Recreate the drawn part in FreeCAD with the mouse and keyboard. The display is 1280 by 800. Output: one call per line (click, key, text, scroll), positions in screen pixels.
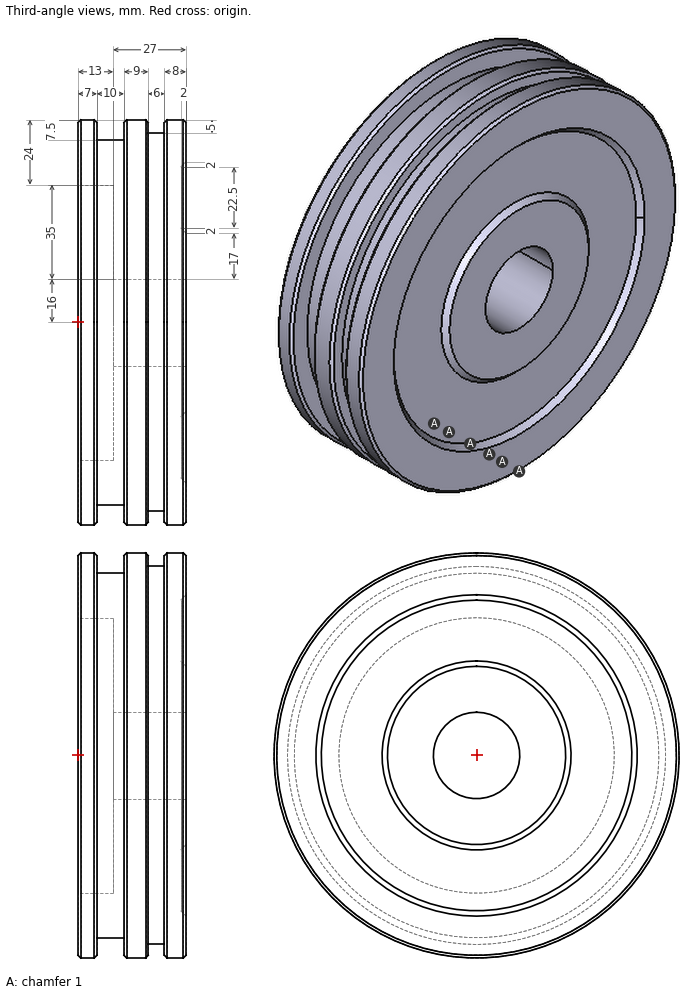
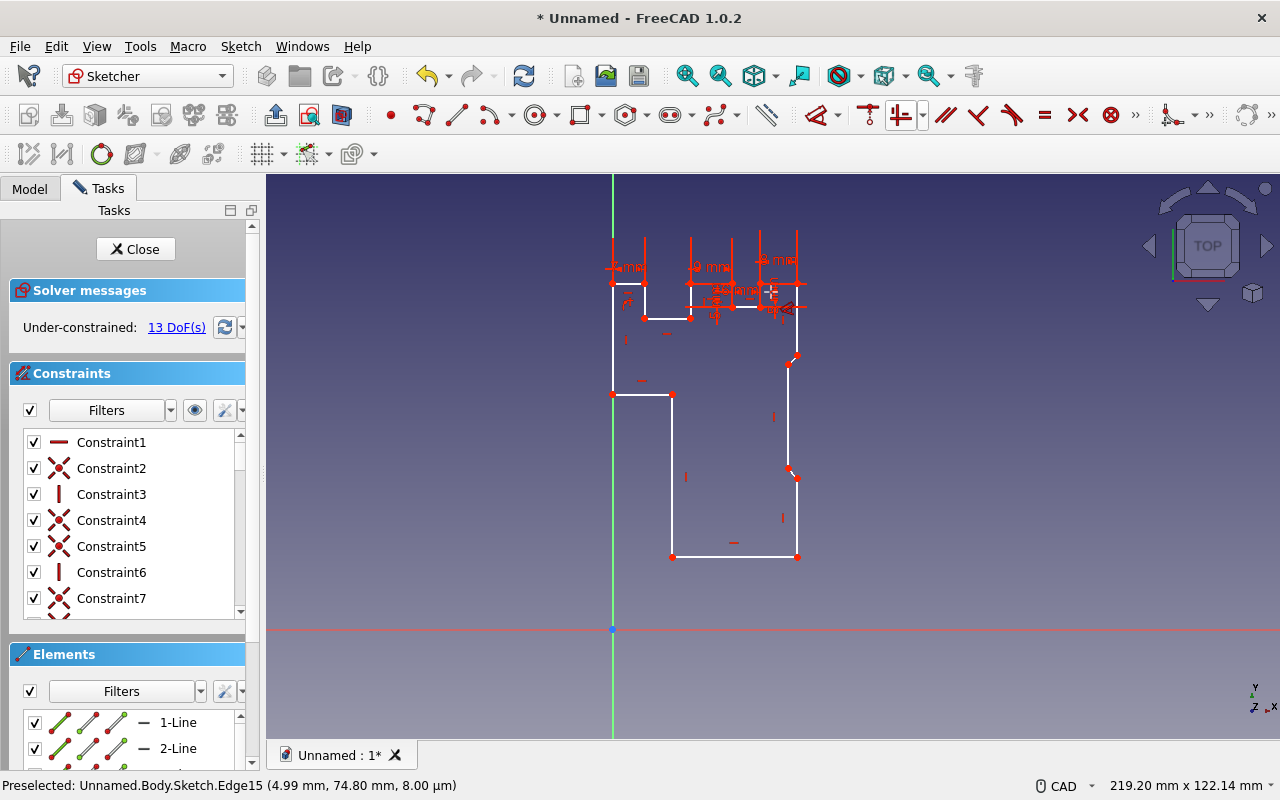
click(710, 557)
click(735, 591)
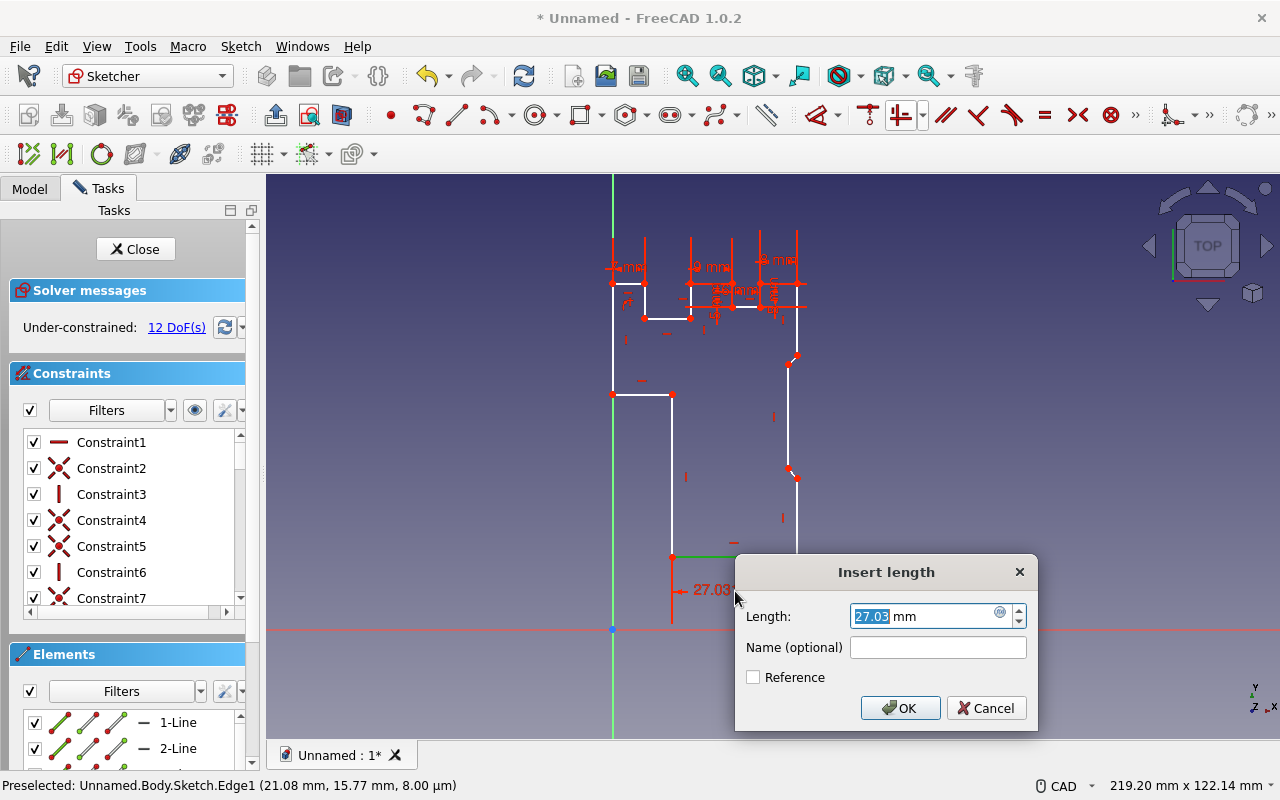
text(27)
key(Return)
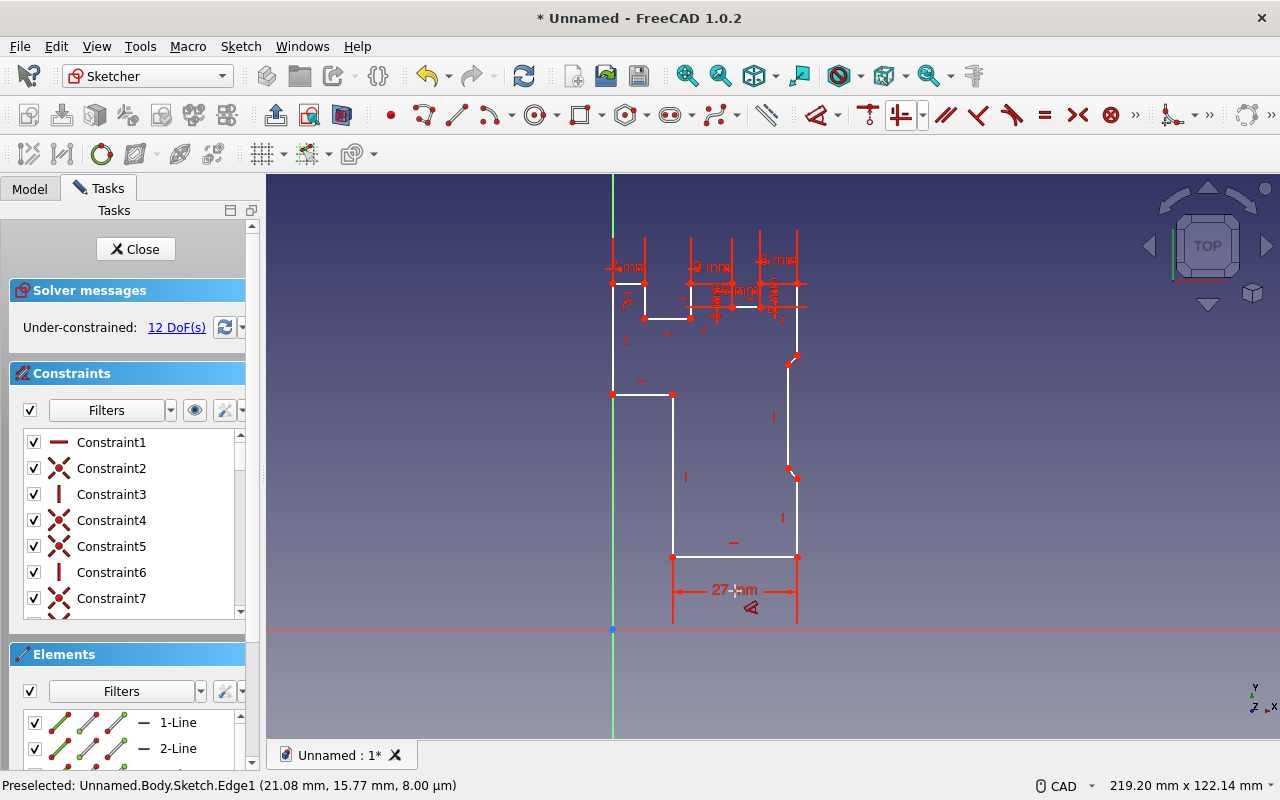
click(797, 534)
click(831, 518)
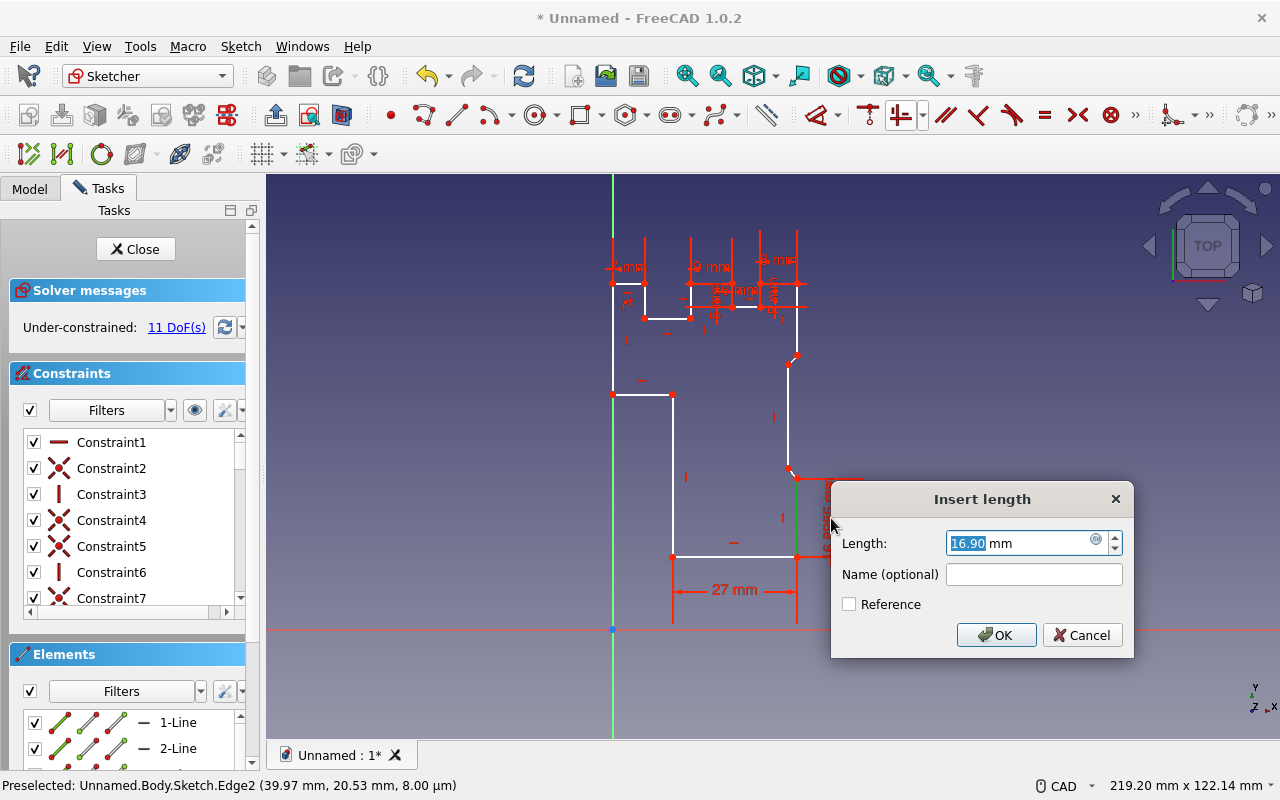
text(17)
key(Return)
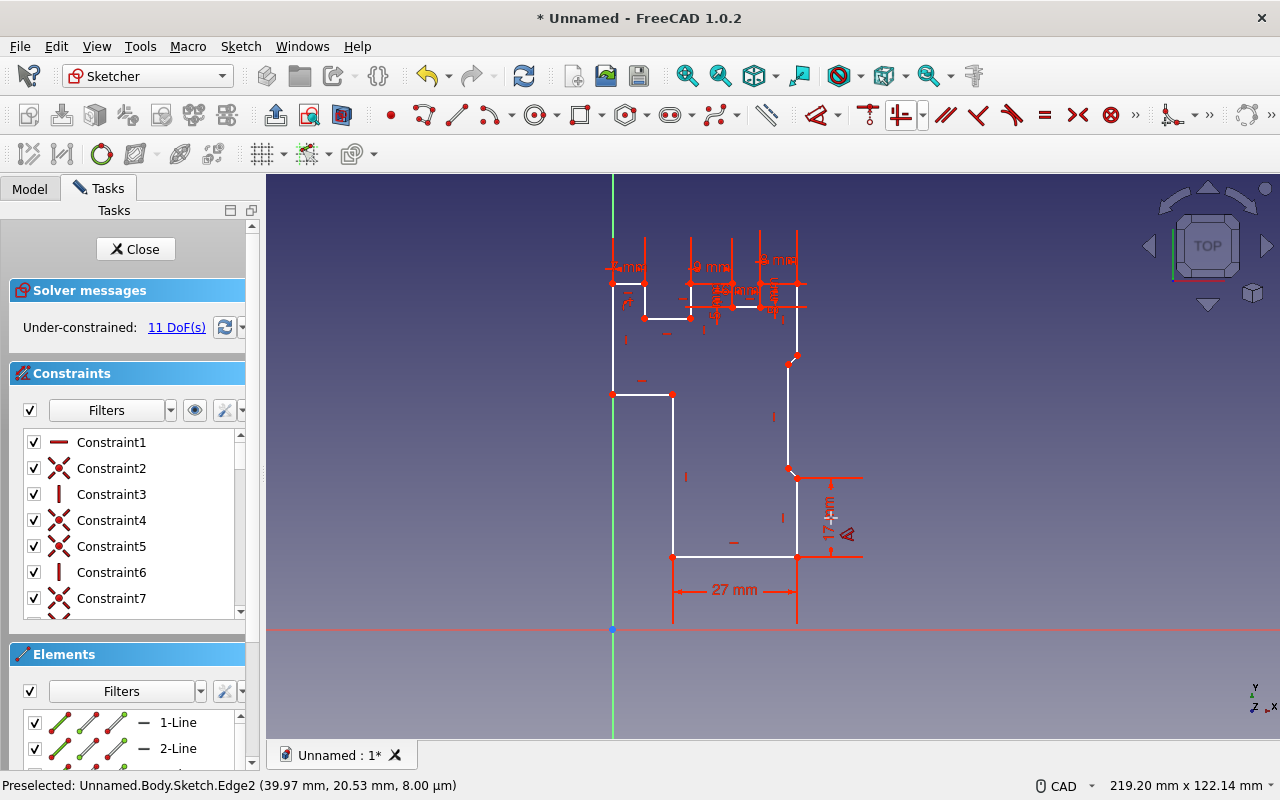
click(677, 319)
click(668, 353)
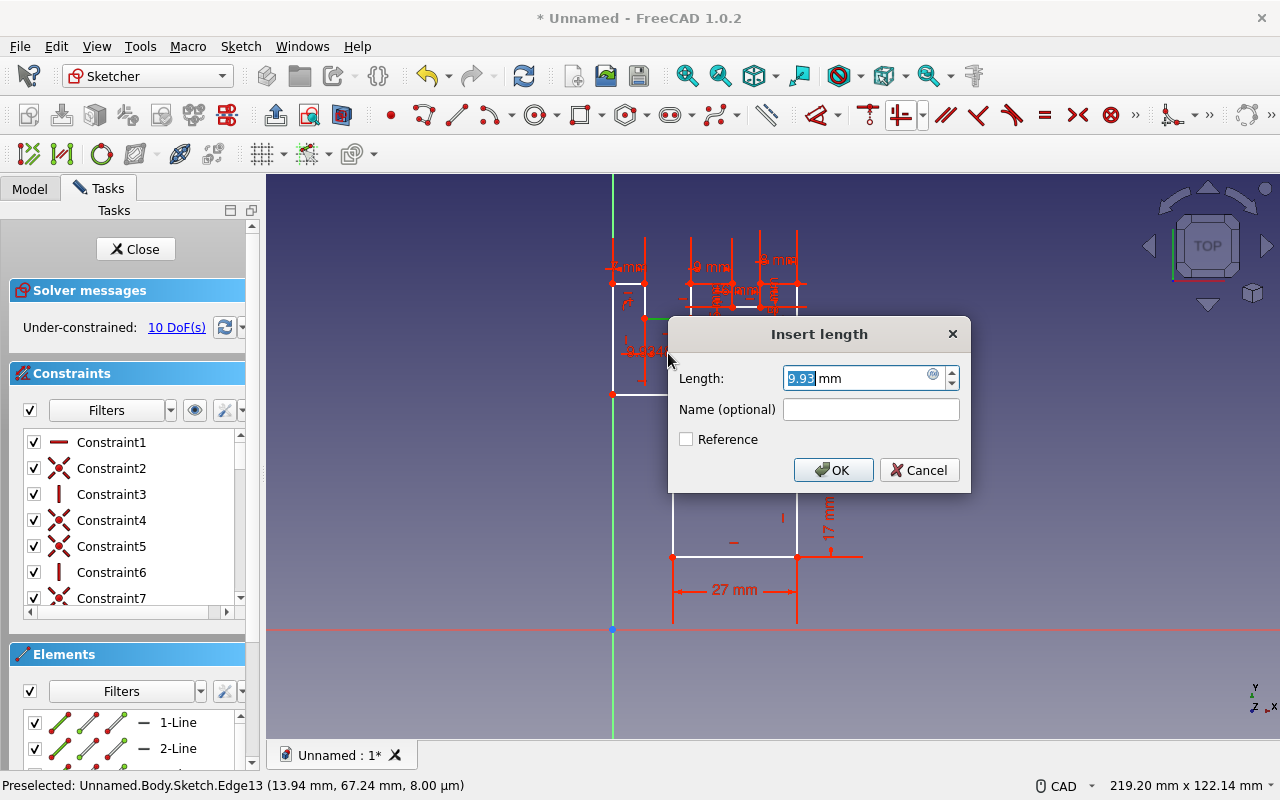
text(10)
key(Return)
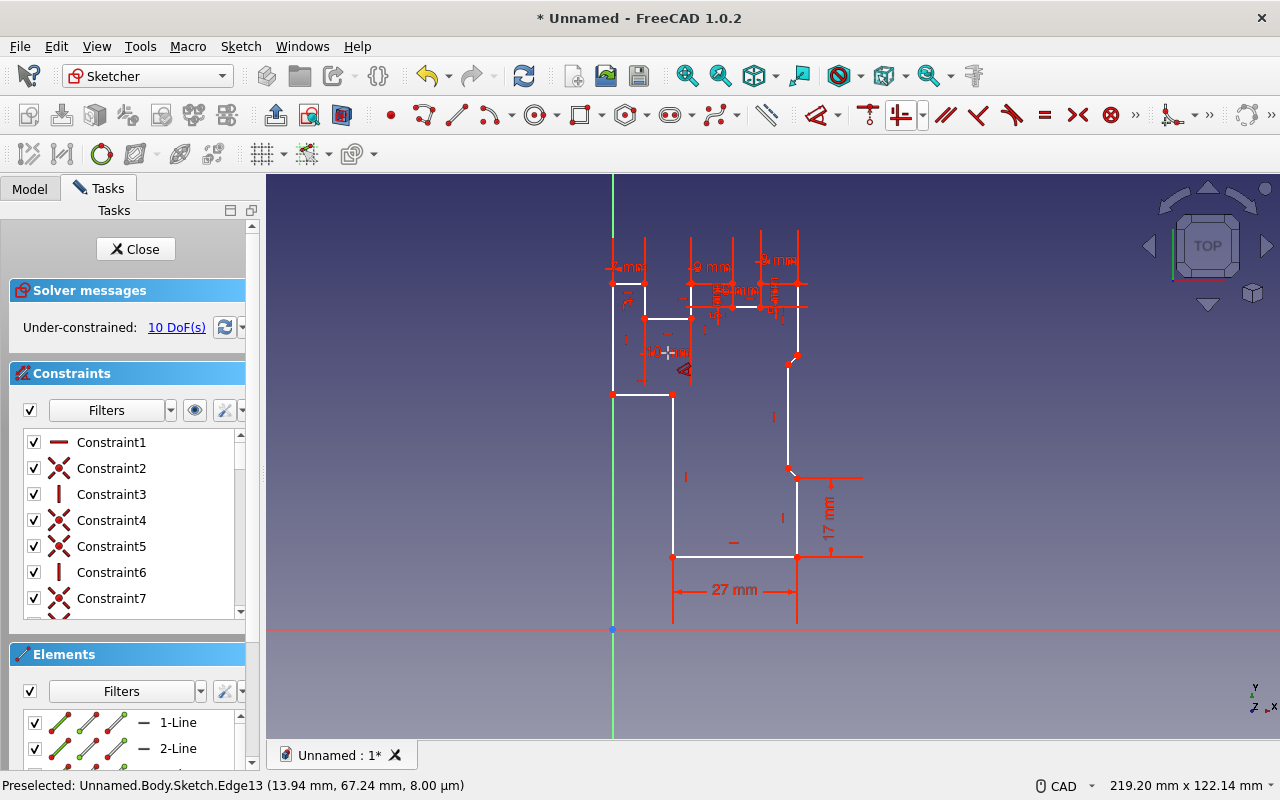
click(613, 317)
click(579, 339)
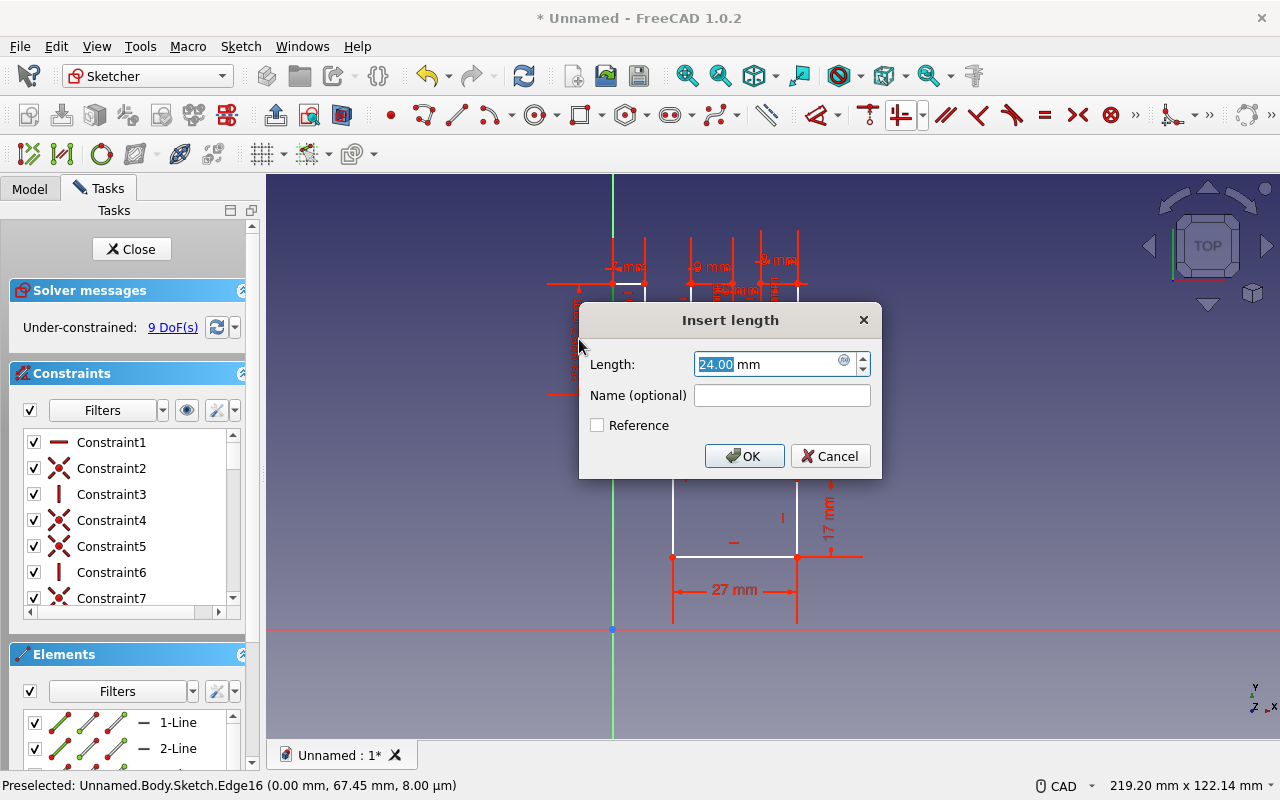
text(24)
key(Return)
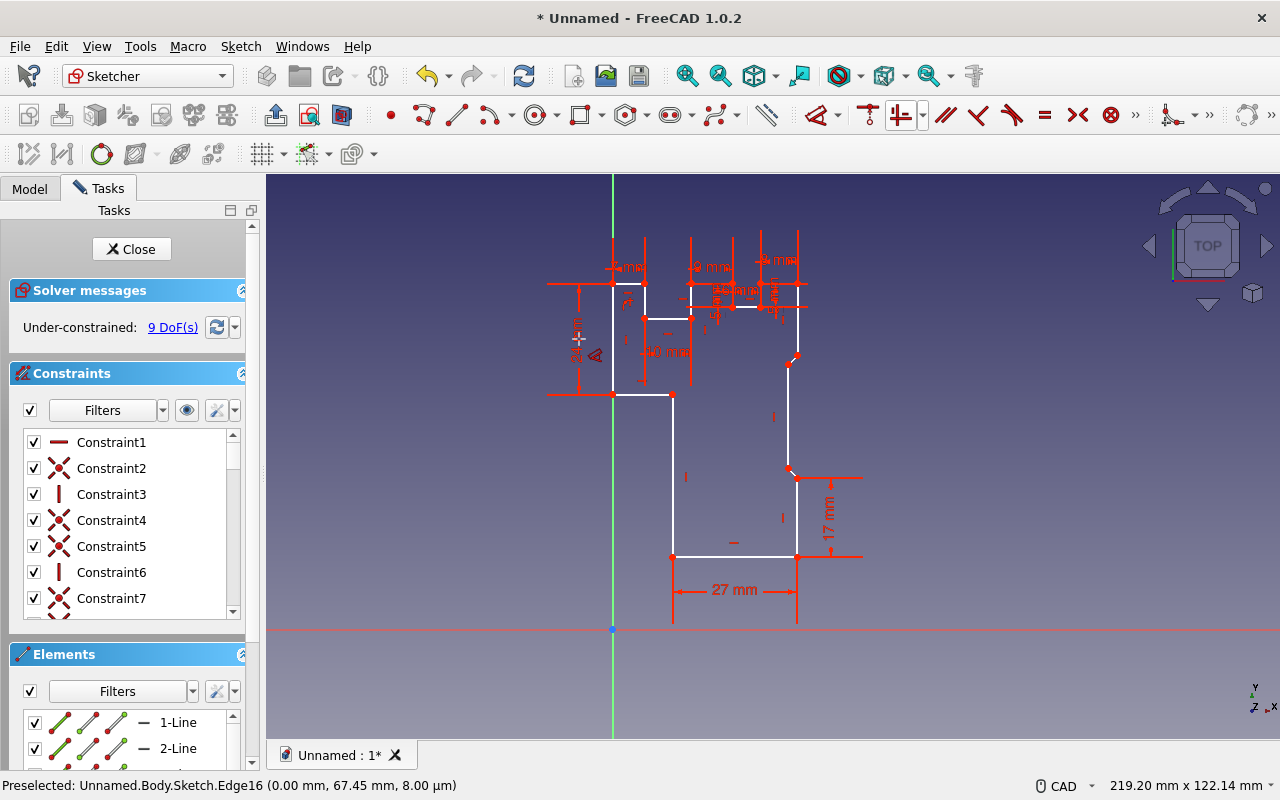
click(631, 395)
click(643, 429)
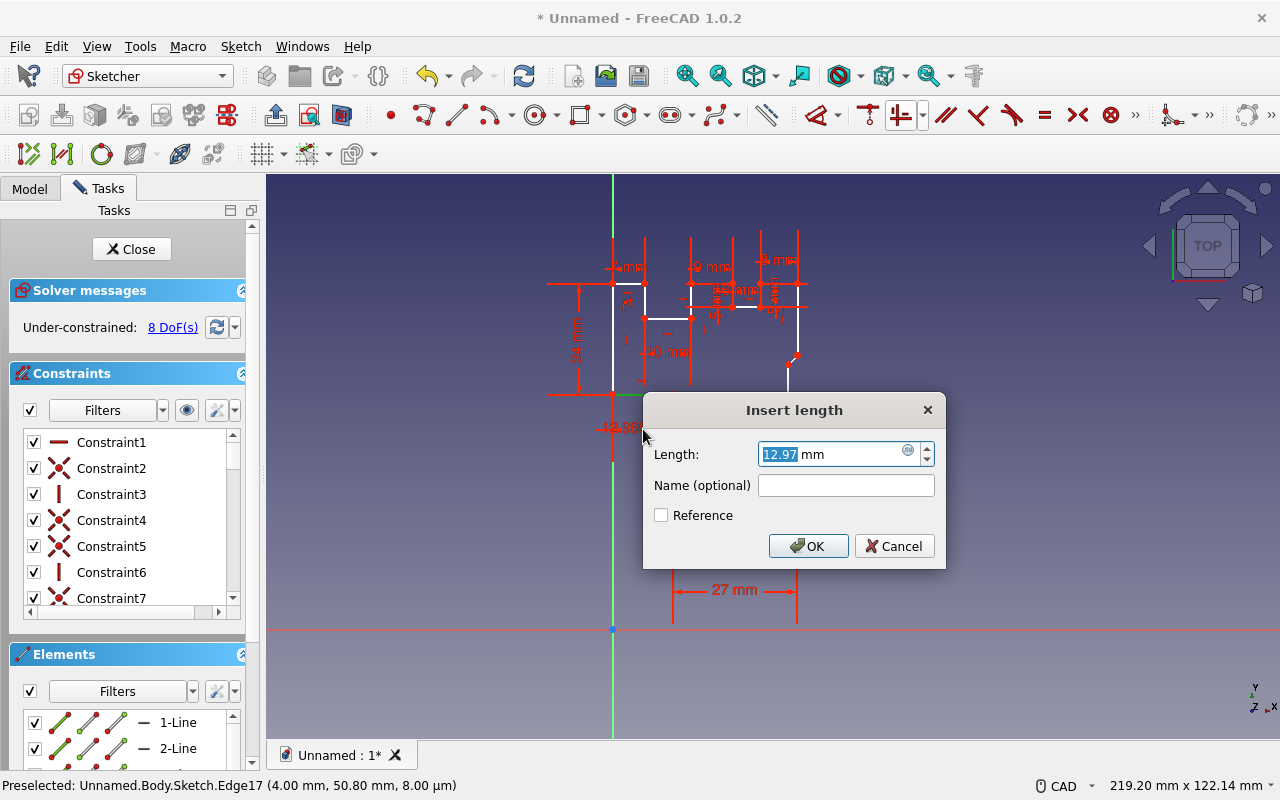
text(13)
key(Return)